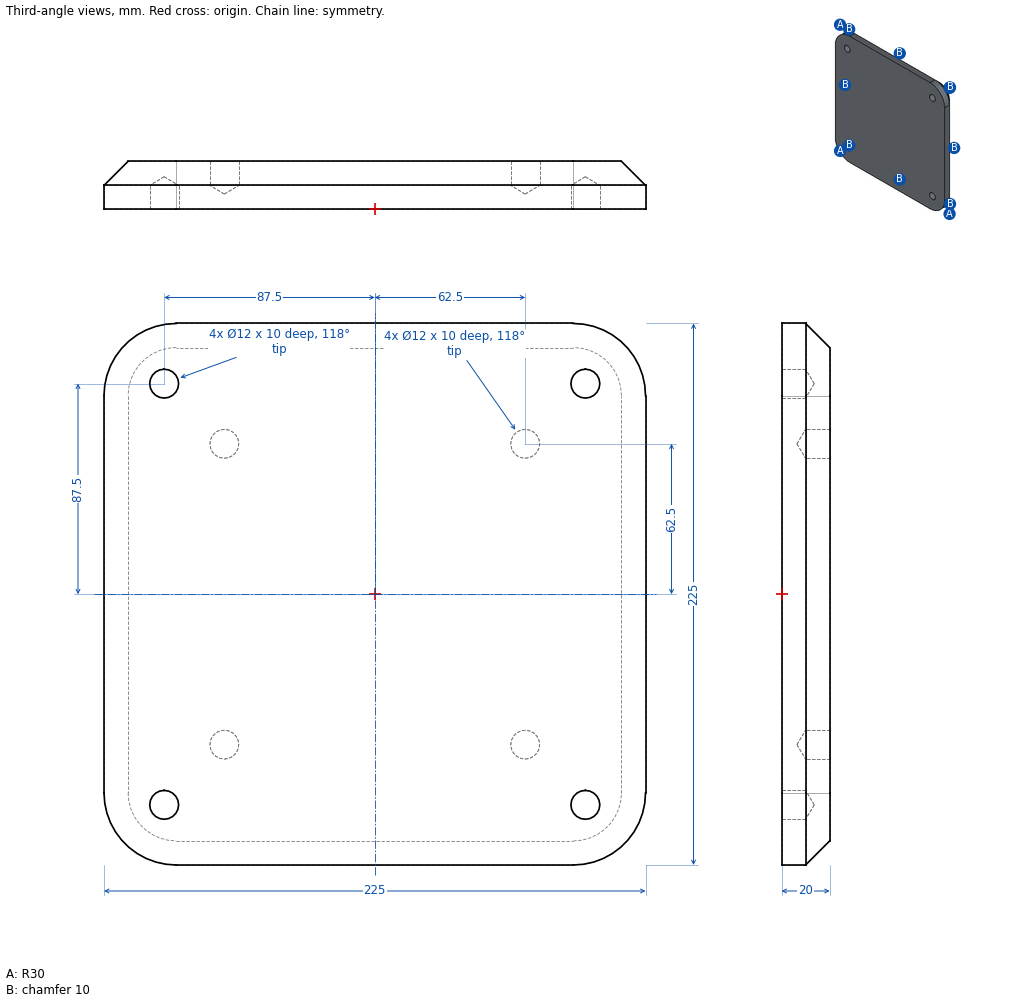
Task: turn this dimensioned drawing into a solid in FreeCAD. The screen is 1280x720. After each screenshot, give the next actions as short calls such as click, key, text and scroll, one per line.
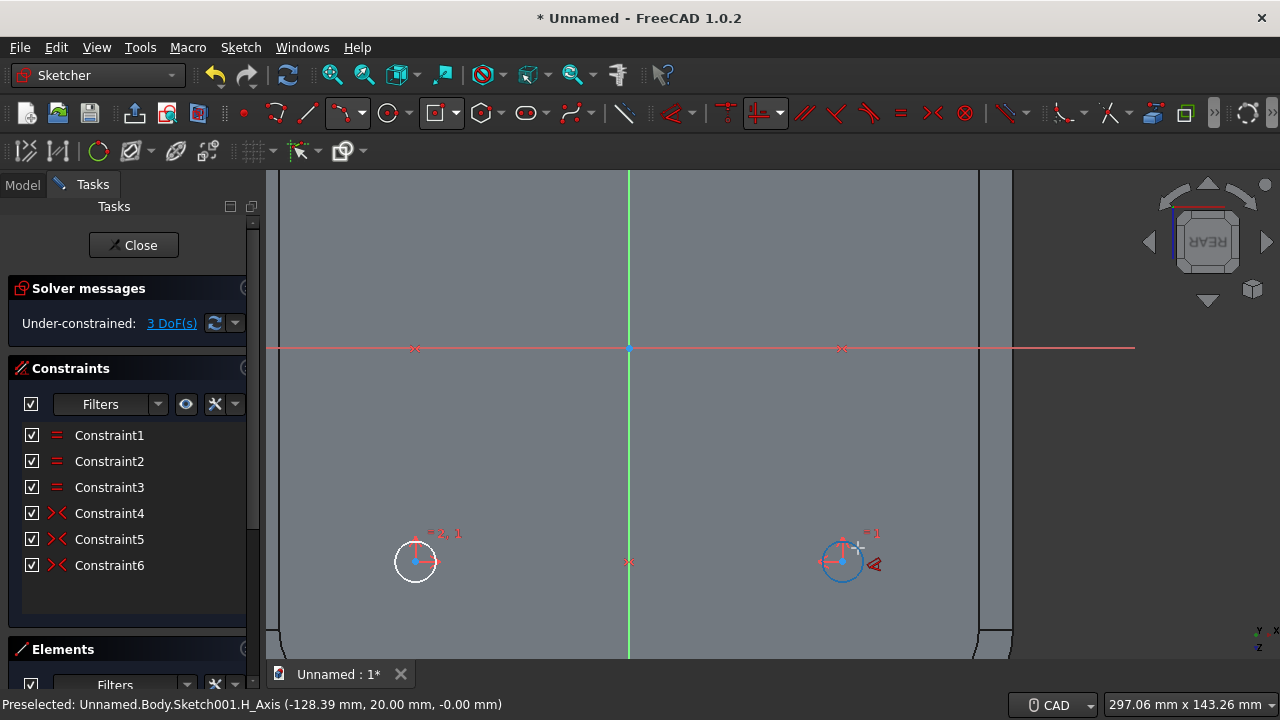
click(857, 547)
click(879, 524)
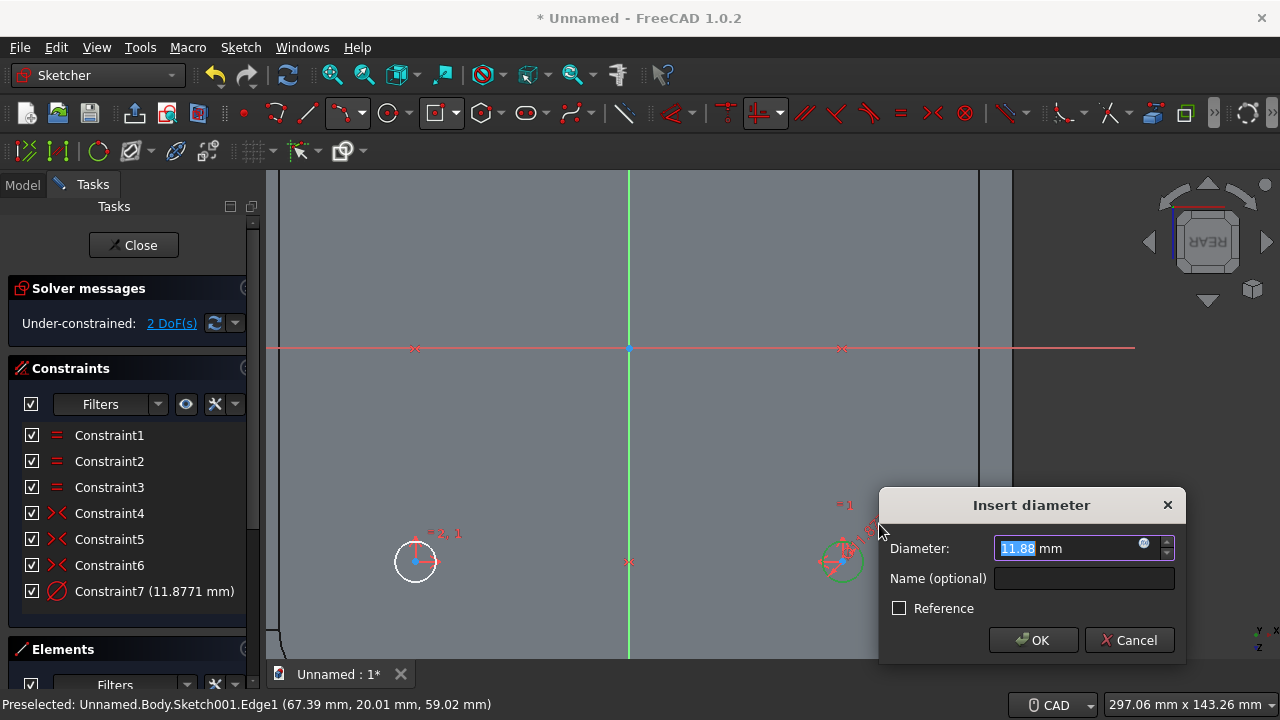
text(12)
key(Return)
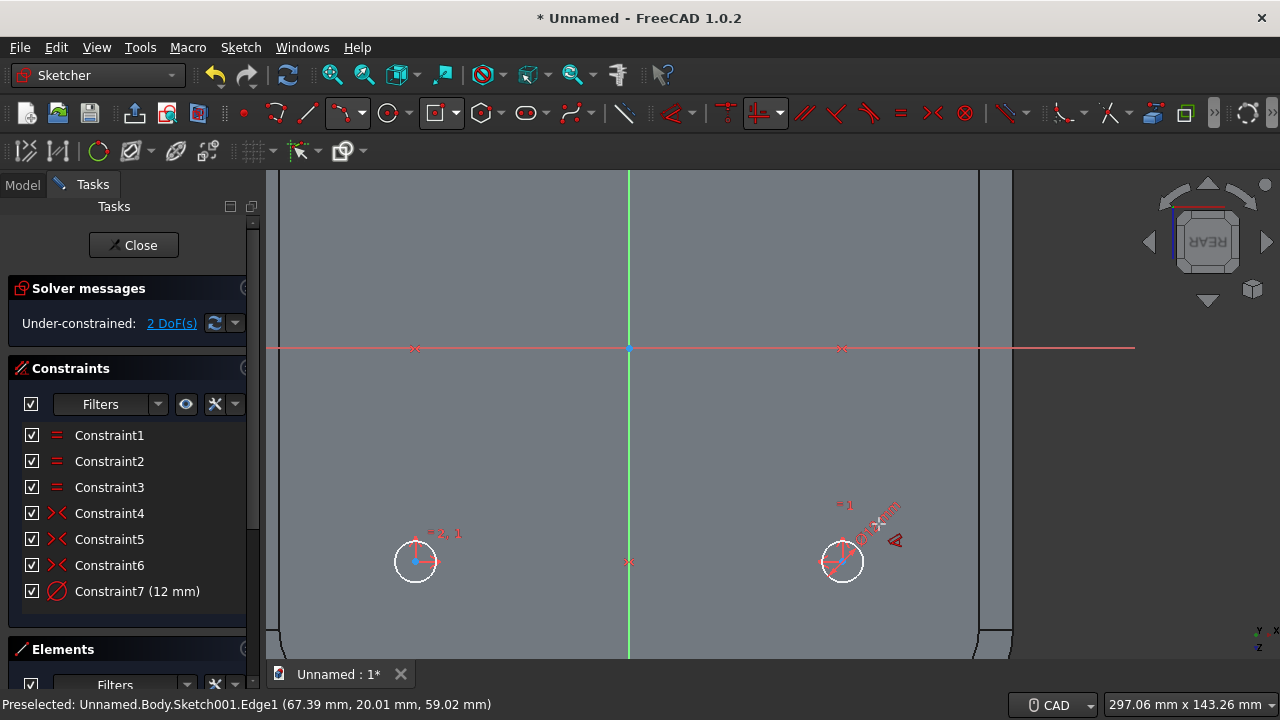
click(843, 562)
click(736, 596)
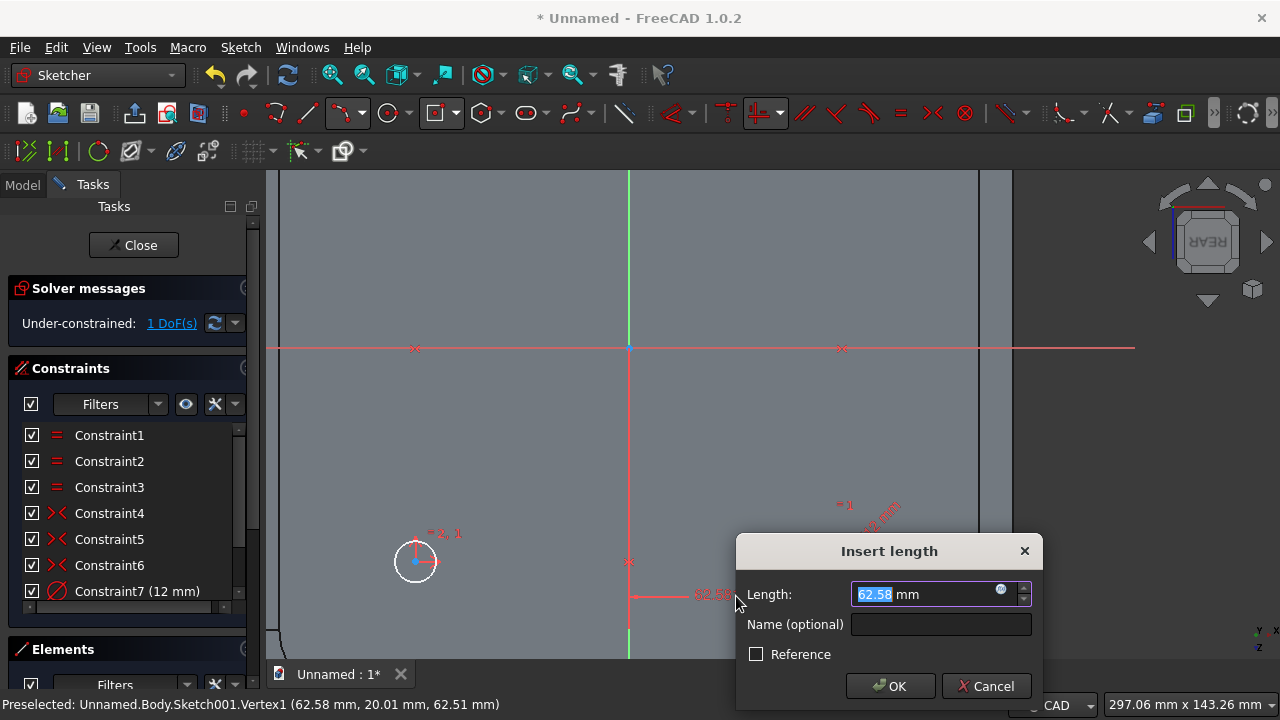
text(62.5)
key(Return)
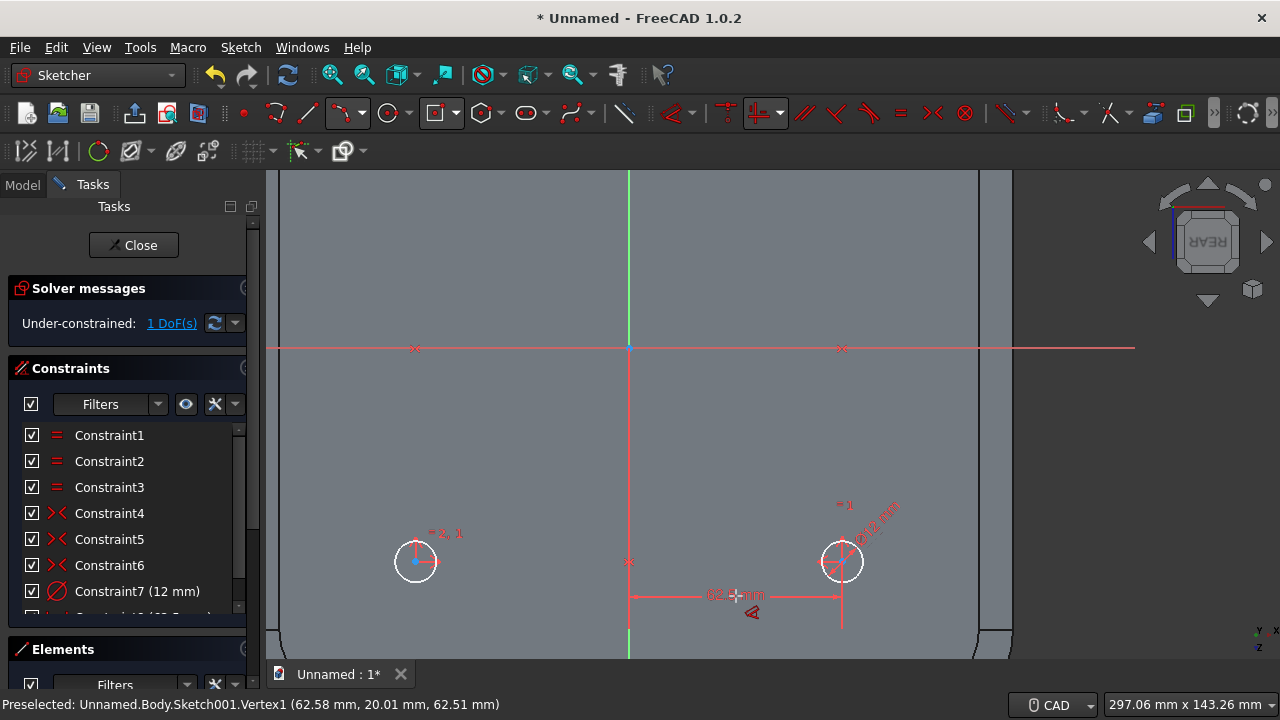
click(842, 562)
click(876, 455)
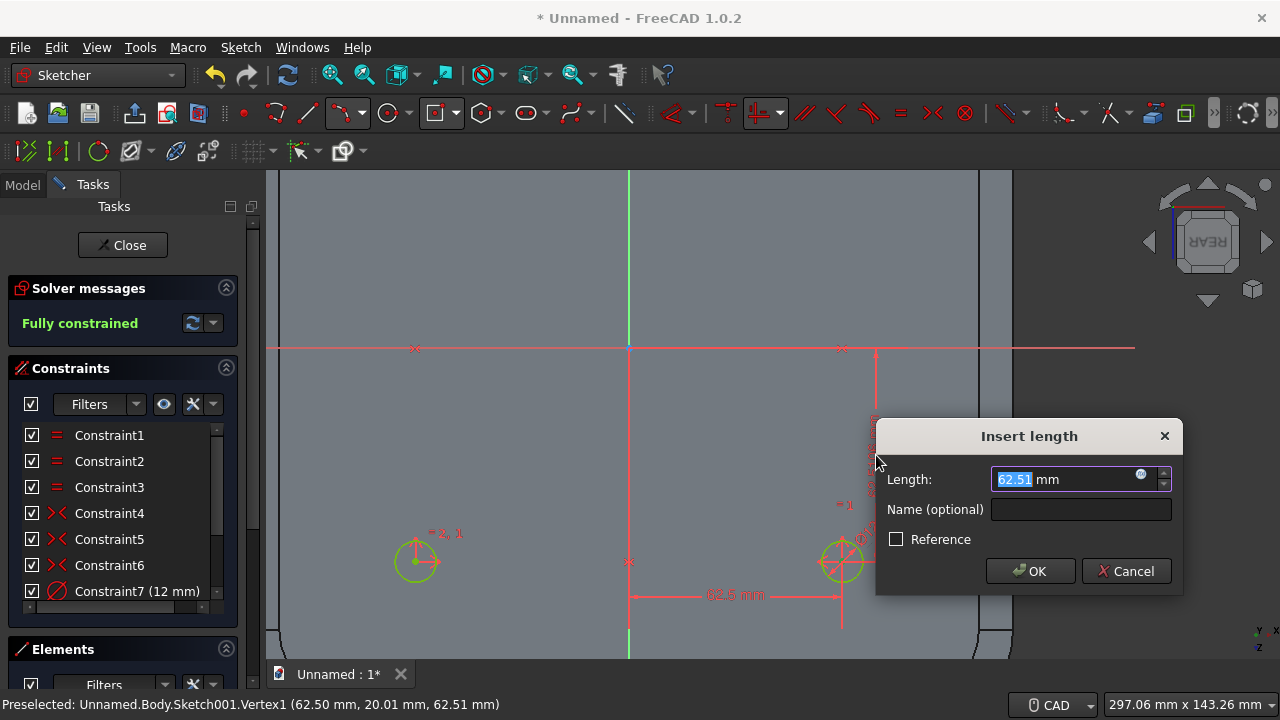
text(62.5)
key(Return)
key(Escape)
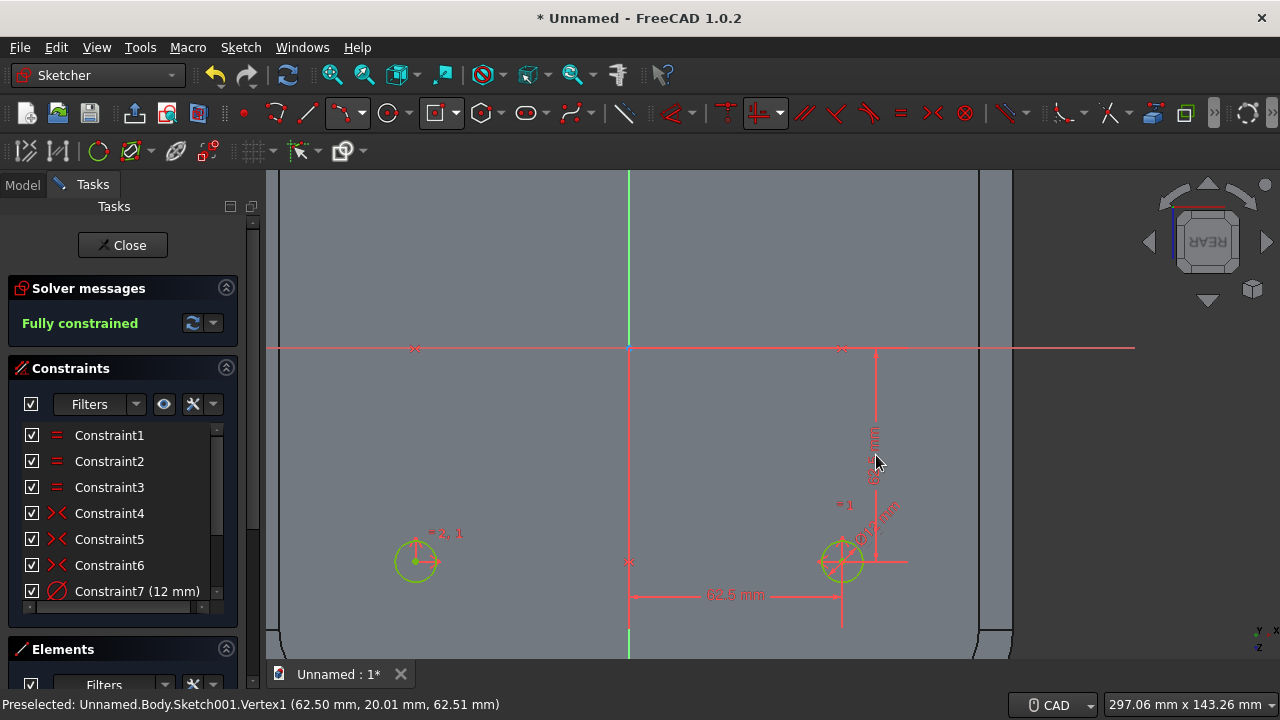
click(123, 245)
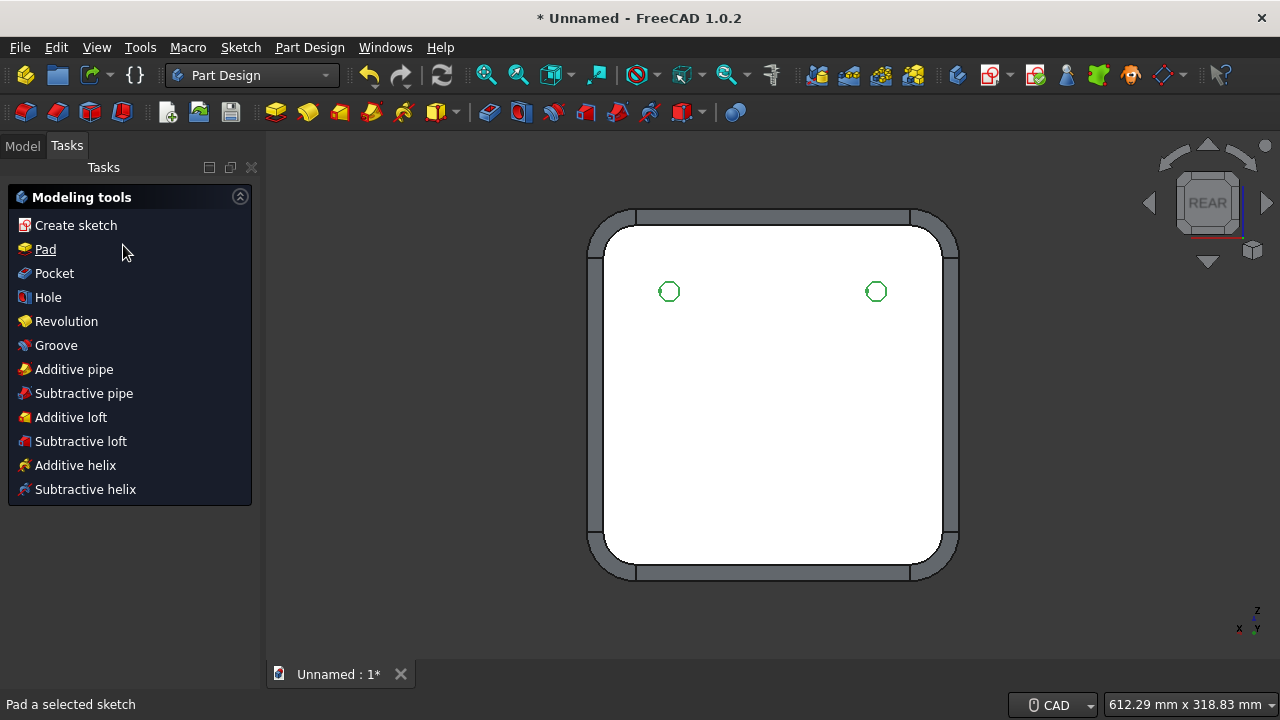
click(522, 112)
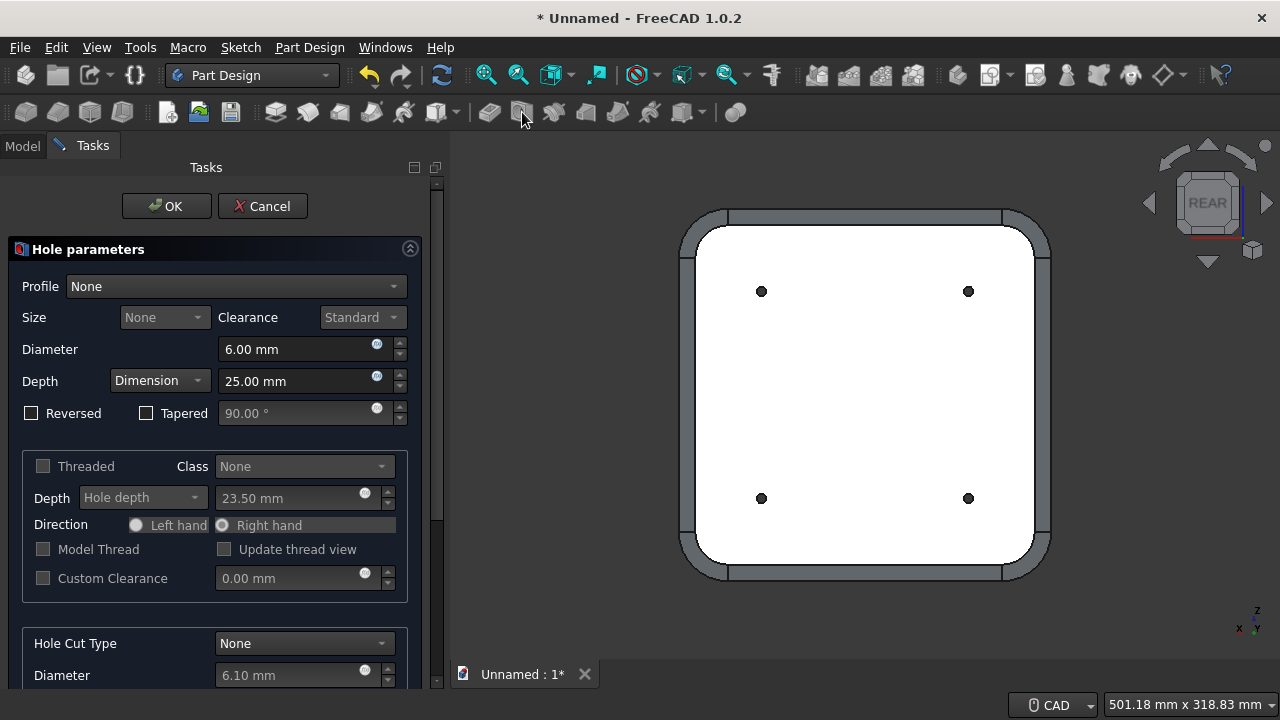
triple_click(305, 349)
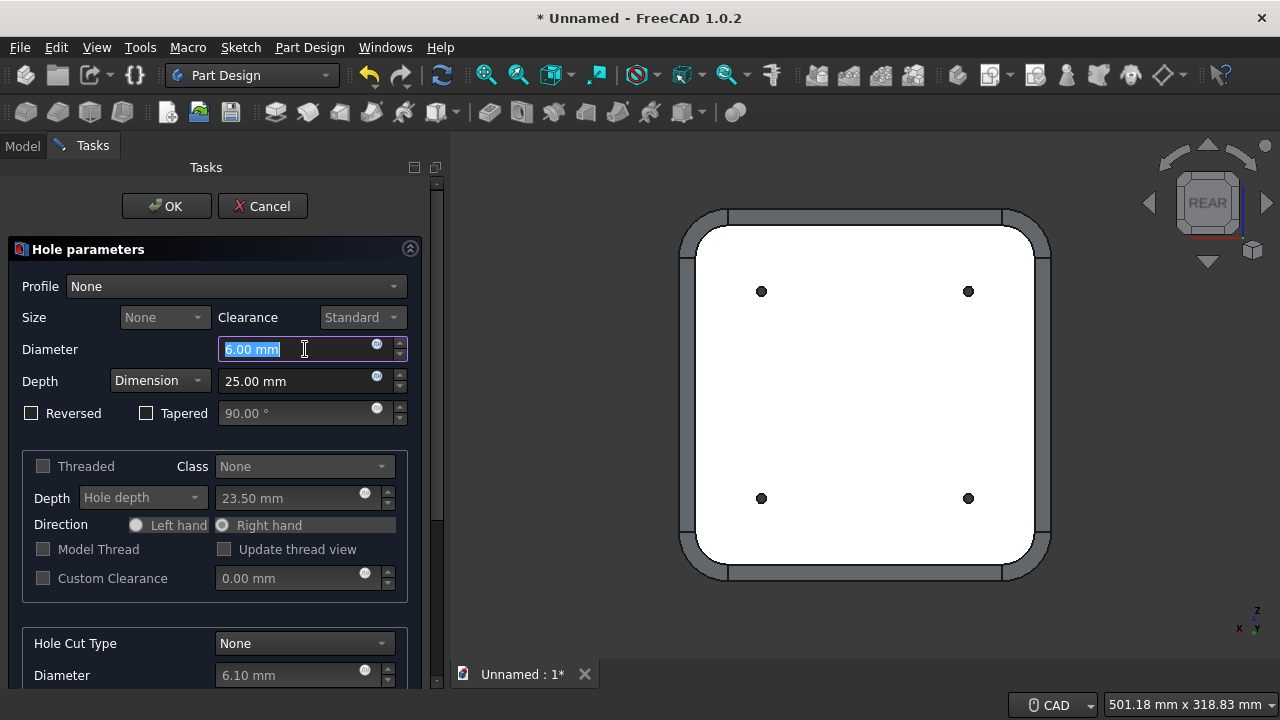
text(12)
key(Tab)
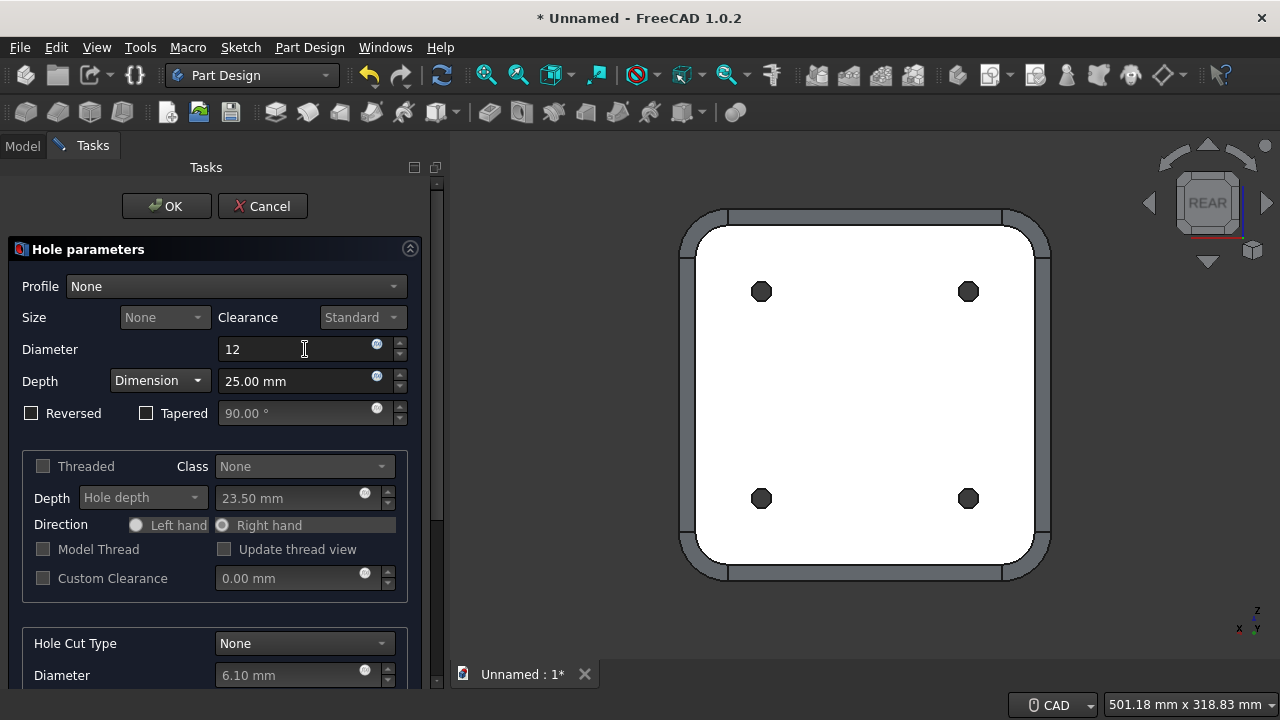
triple_click(305, 381)